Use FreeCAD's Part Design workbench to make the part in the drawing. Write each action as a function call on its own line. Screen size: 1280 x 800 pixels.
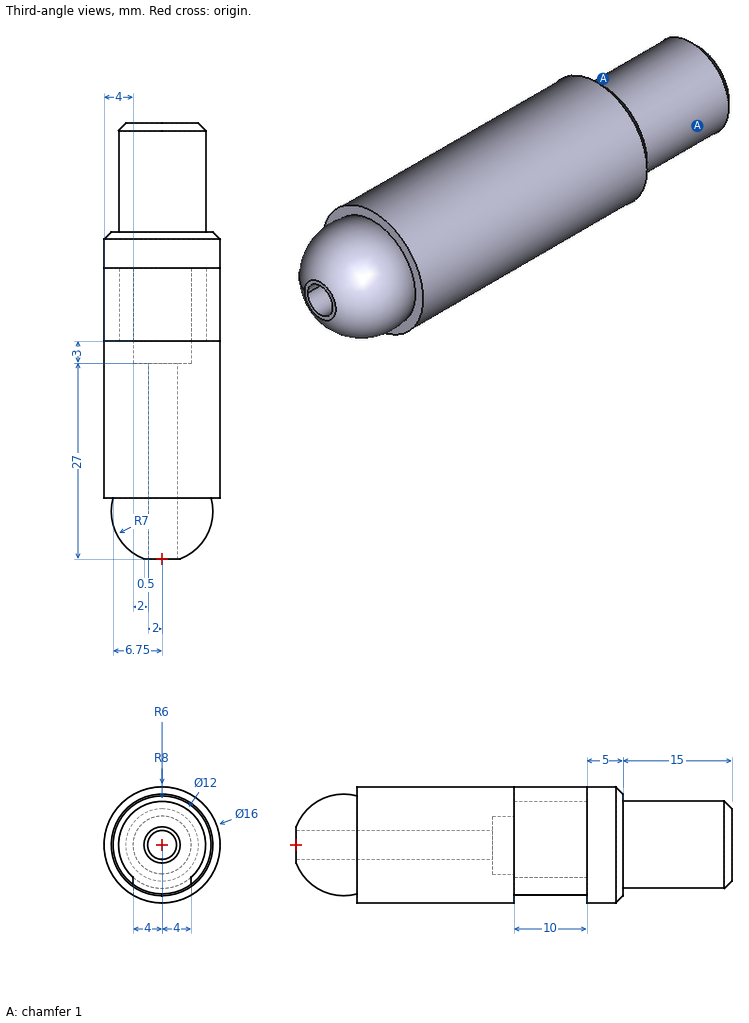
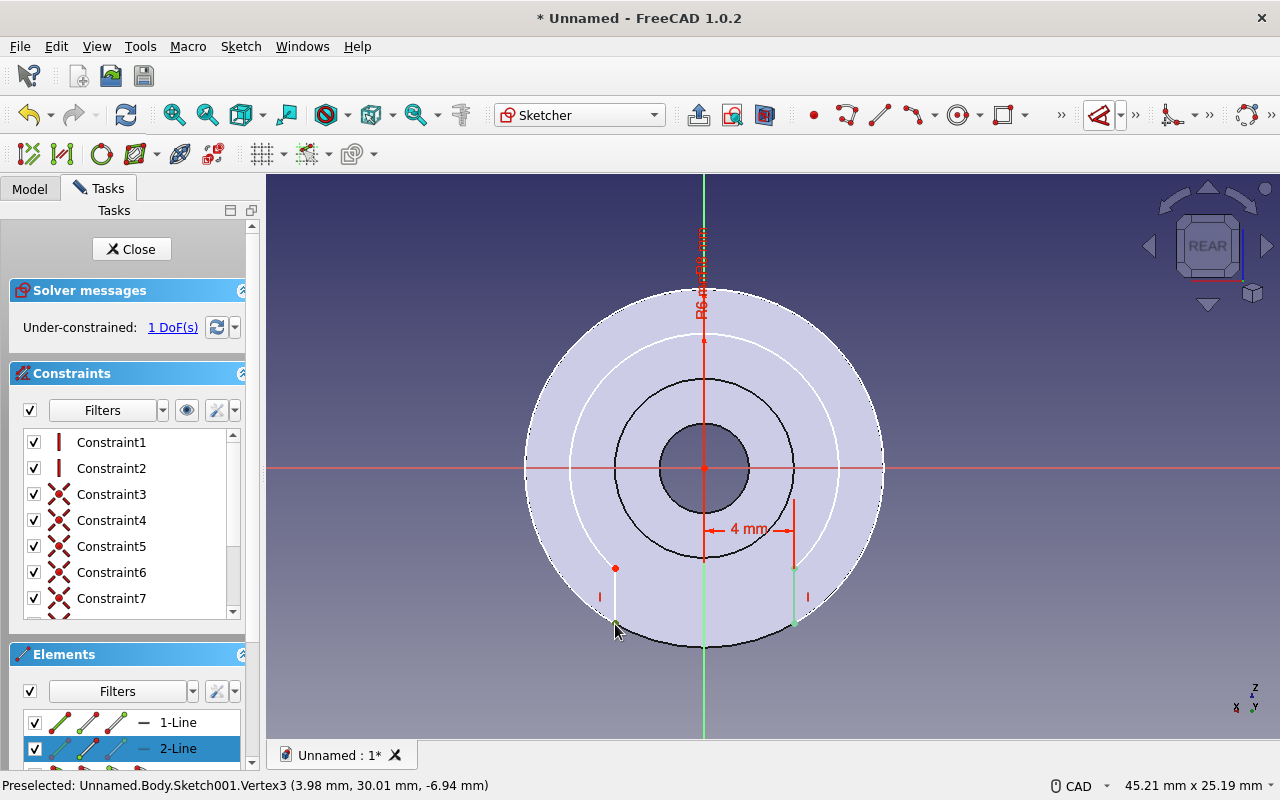
key(l)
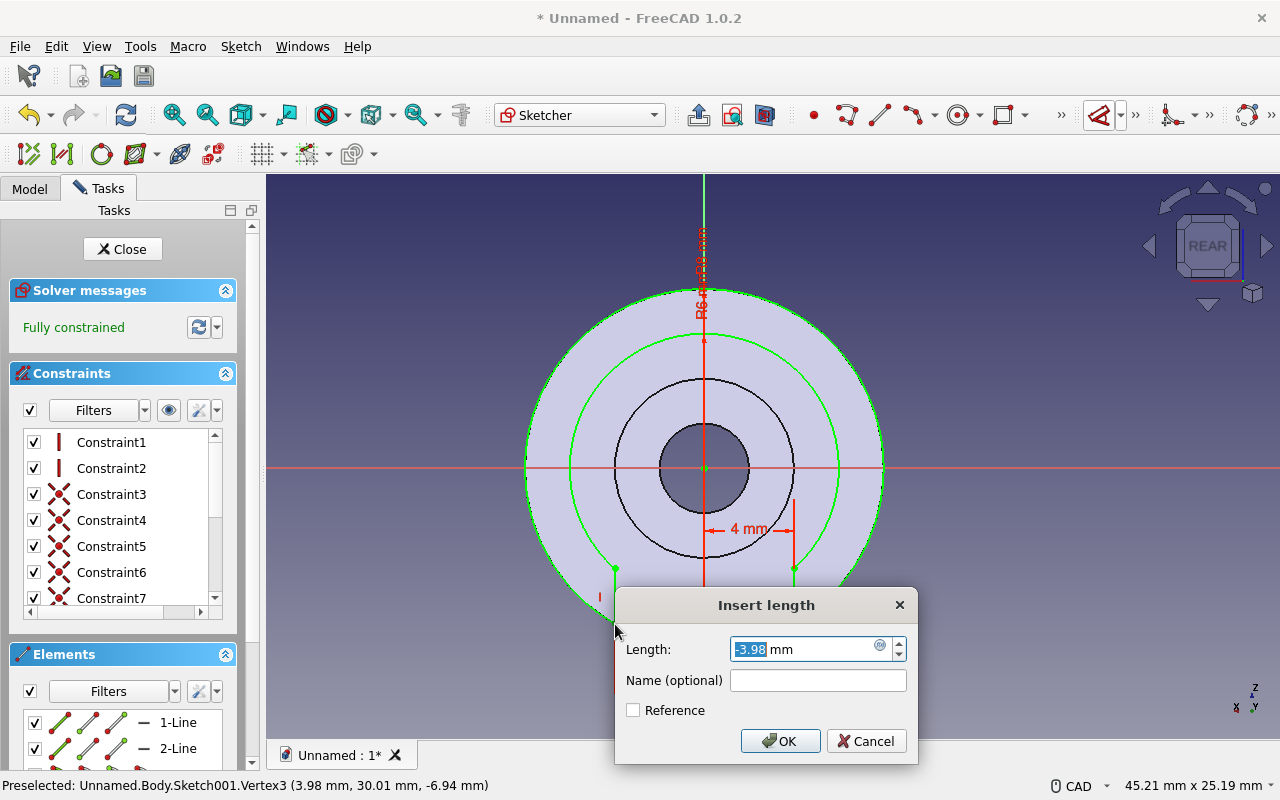
text(-4)
key(Return)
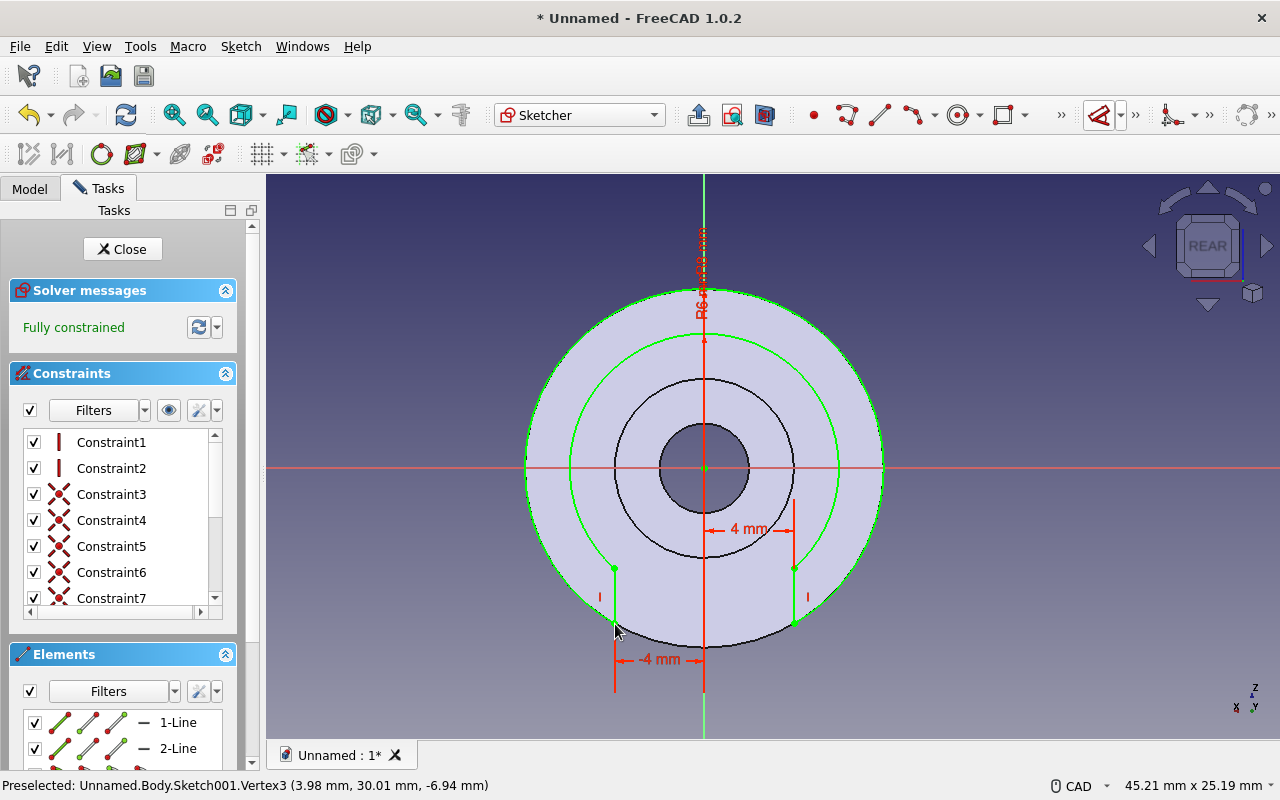
click(123, 249)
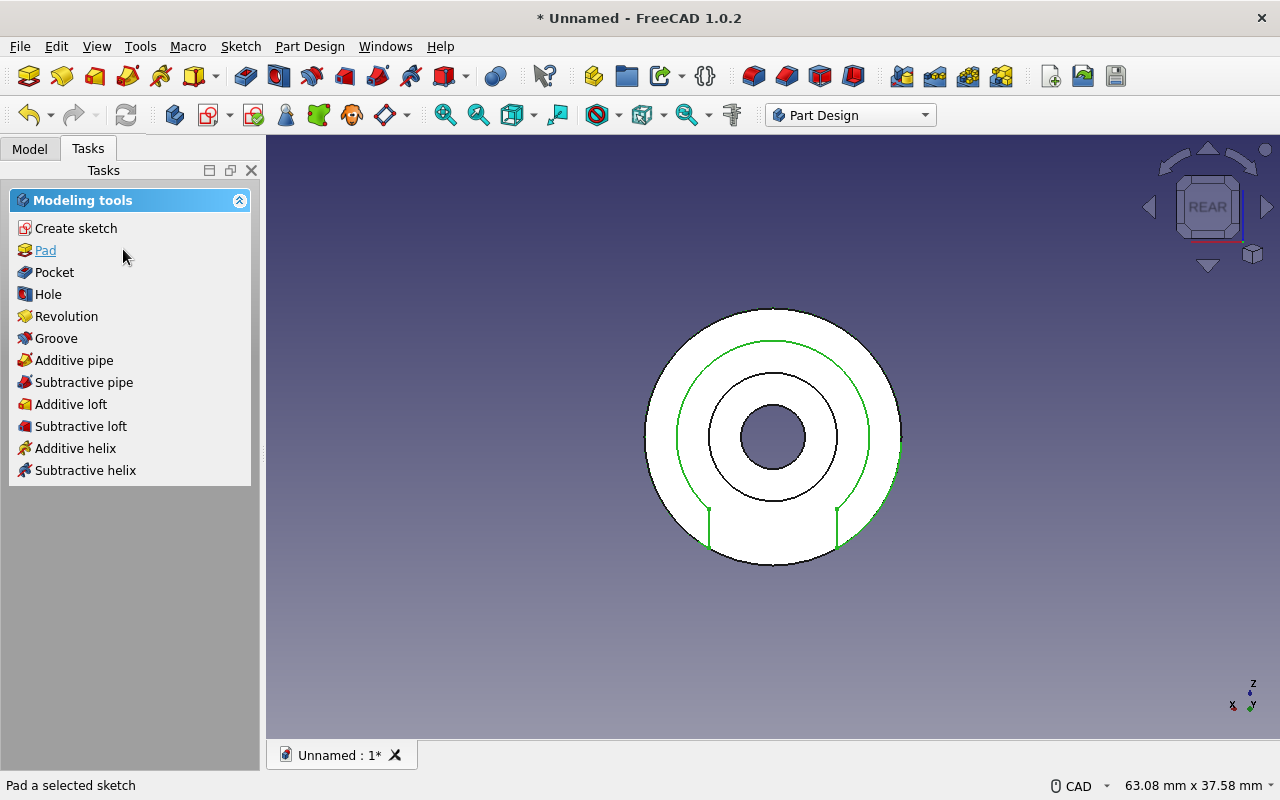
click(29, 76)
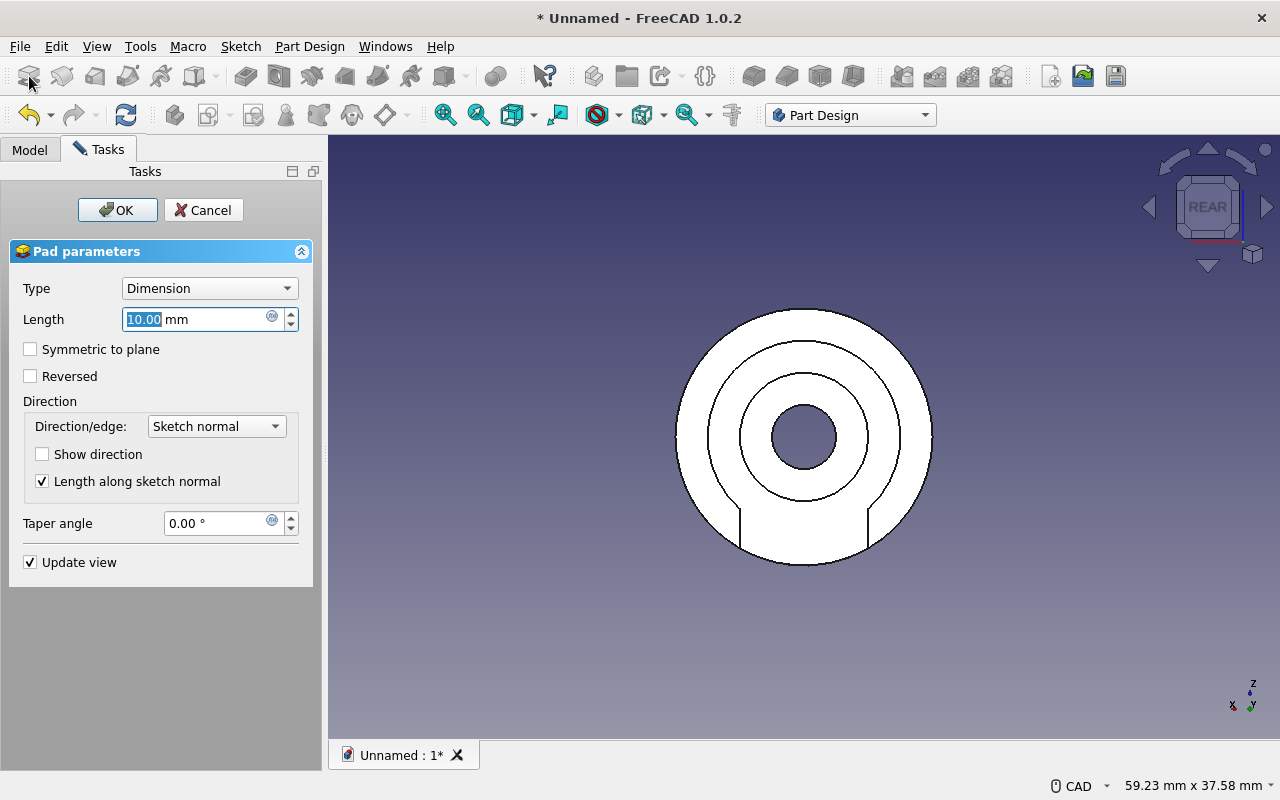
text(10)
key(Tab)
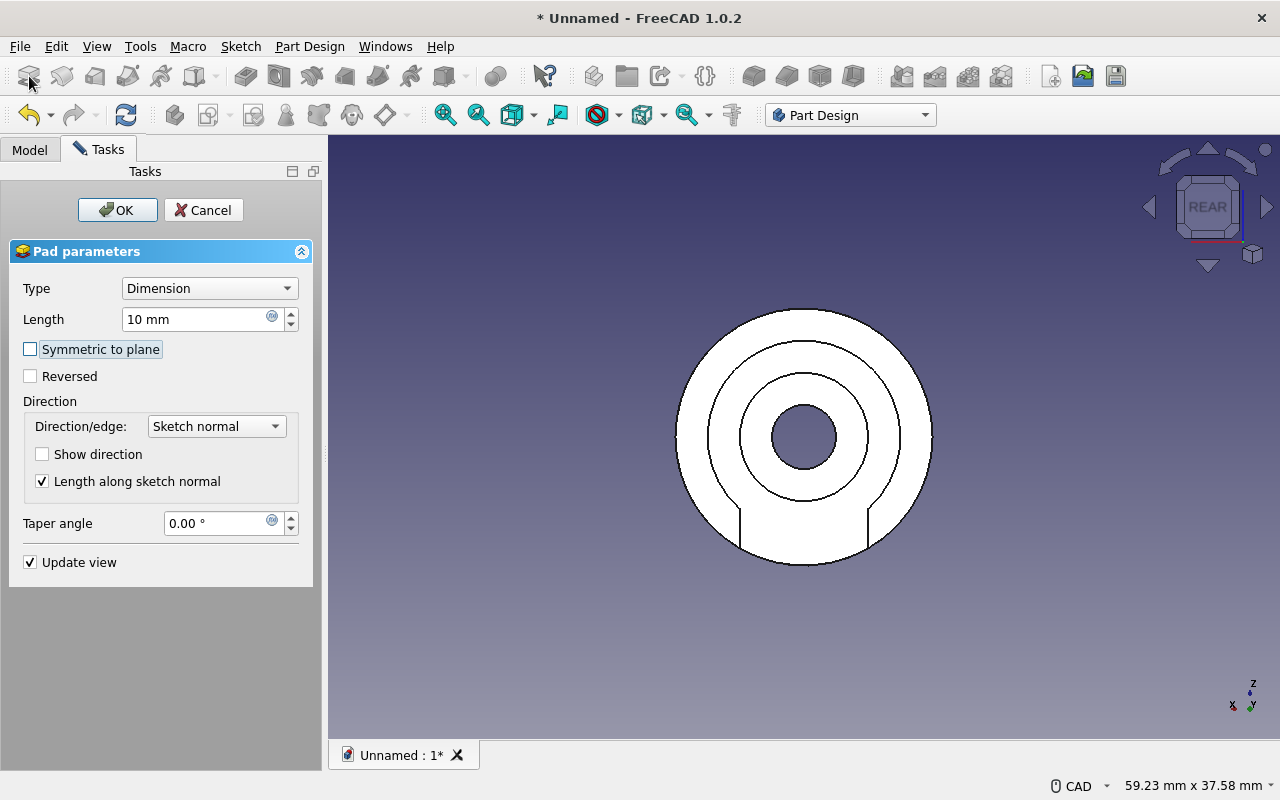
click(118, 210)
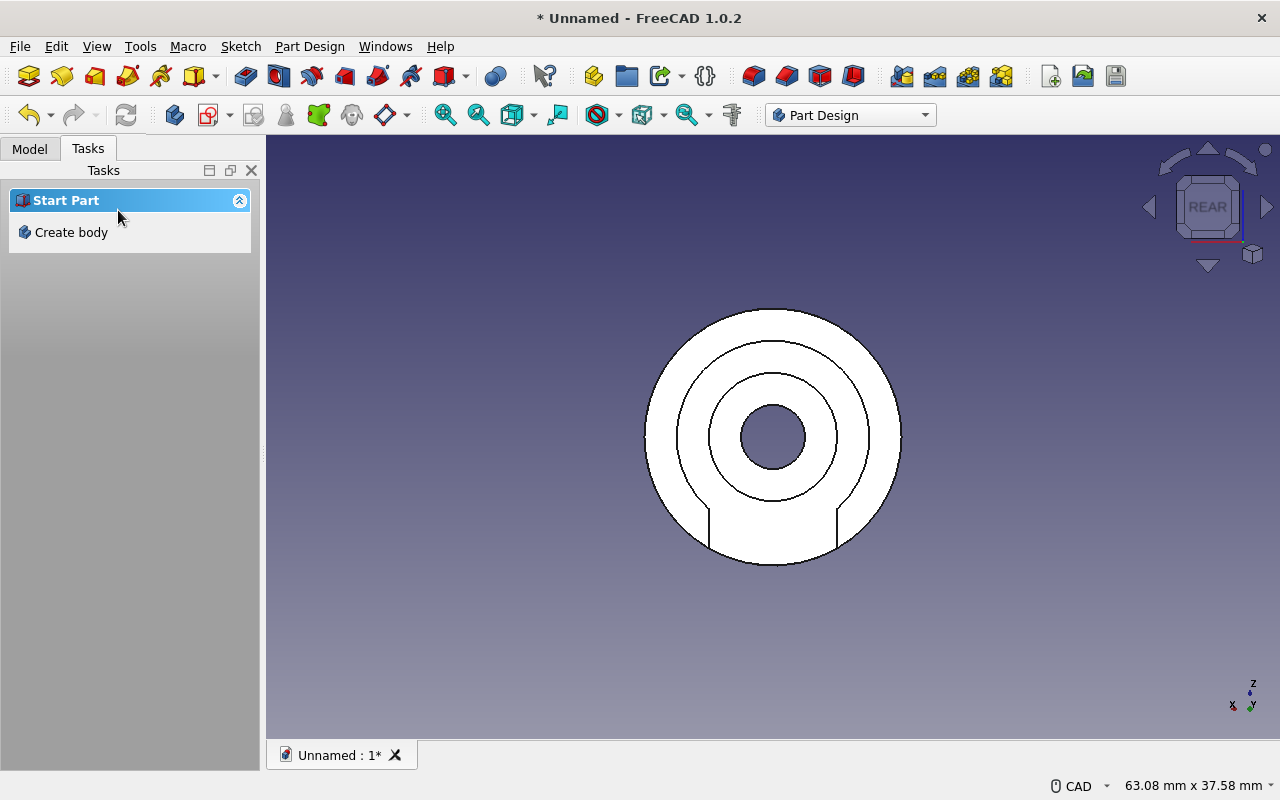
click(446, 116)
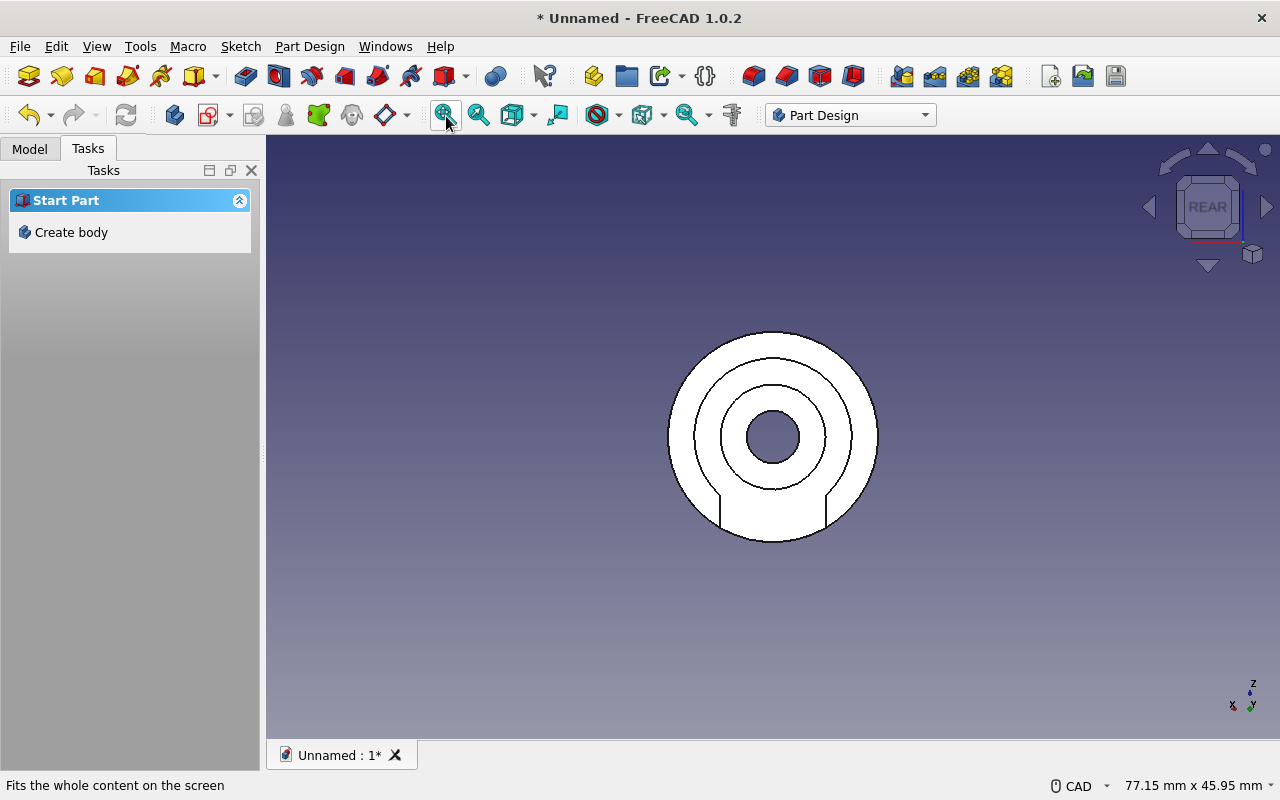
click(863, 457)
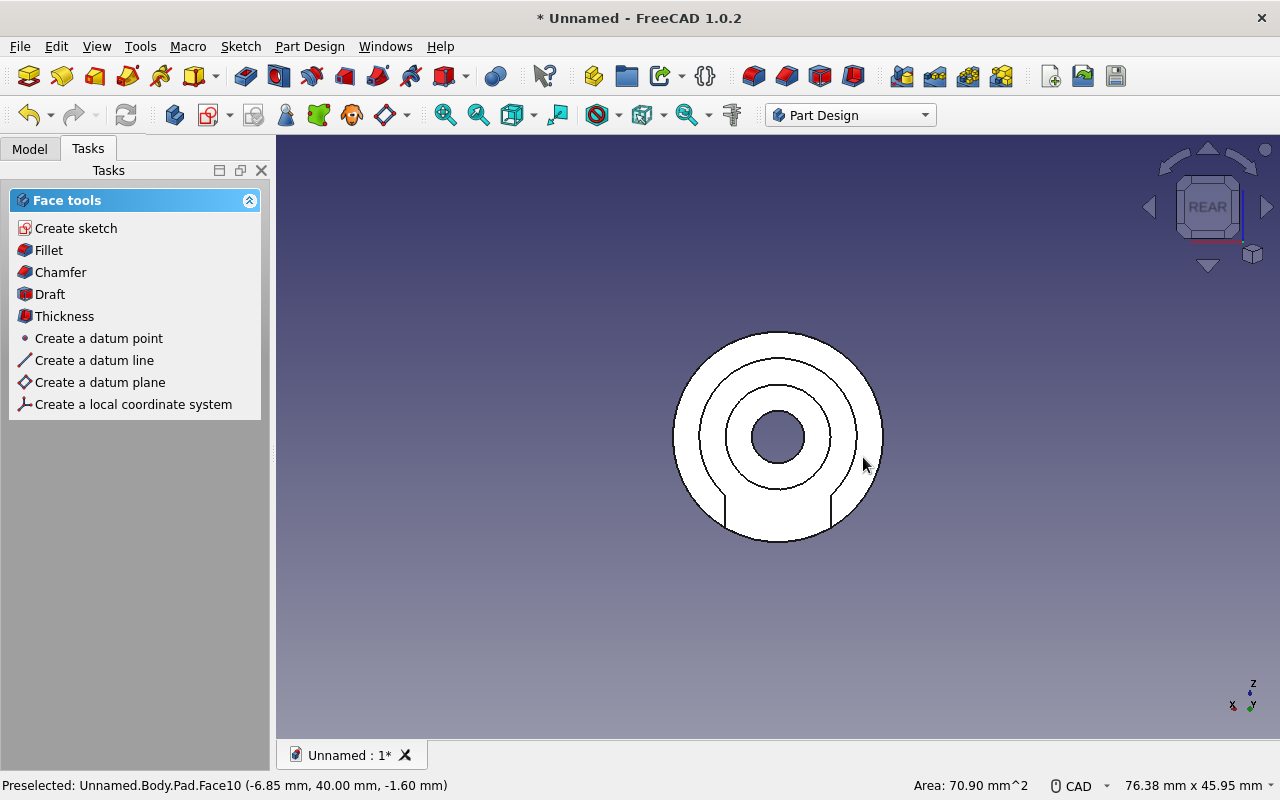
click(208, 116)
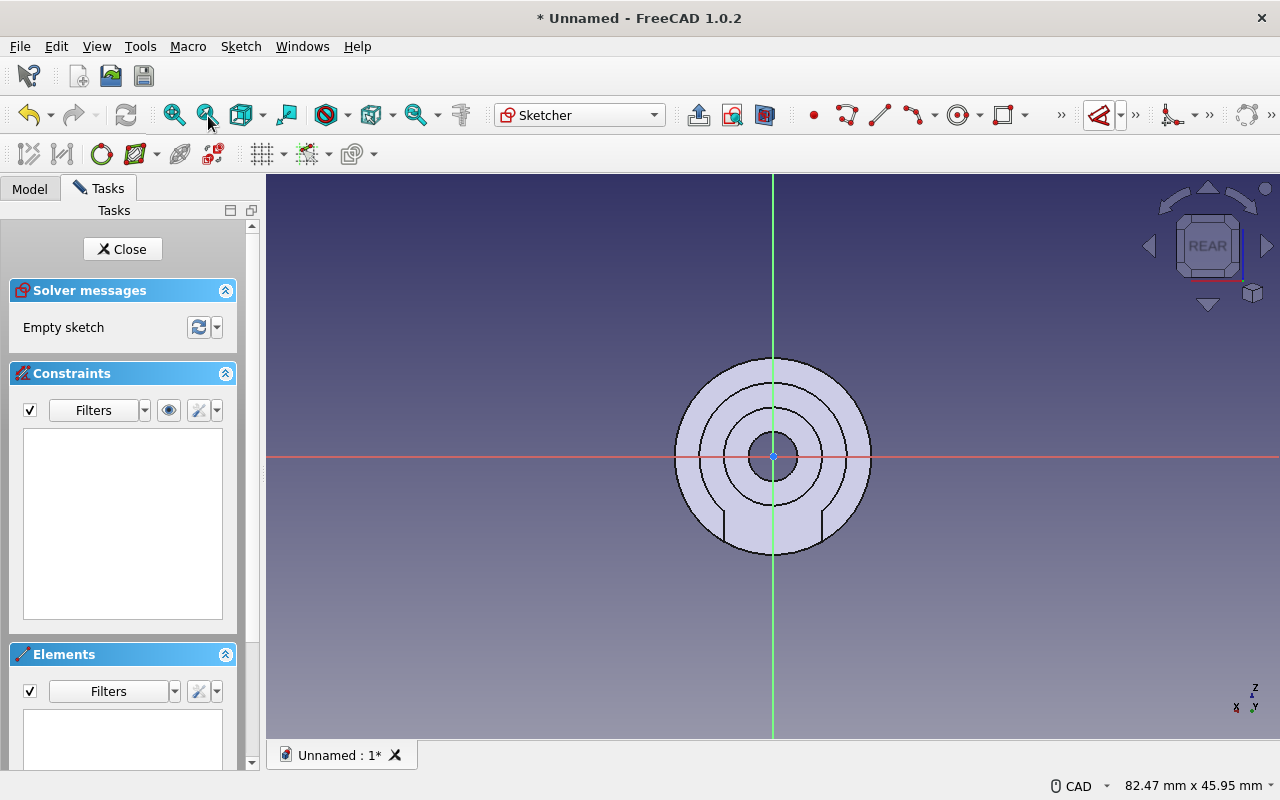
scroll(856, 457, up, 3)